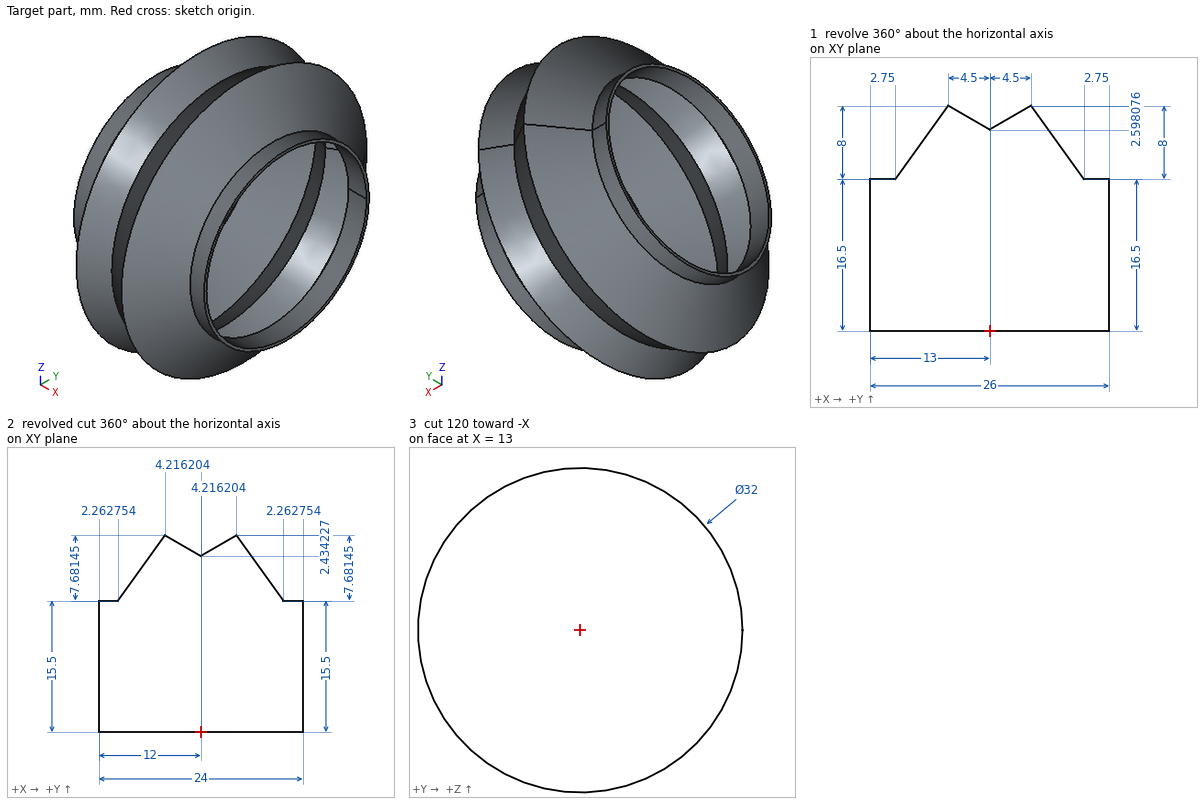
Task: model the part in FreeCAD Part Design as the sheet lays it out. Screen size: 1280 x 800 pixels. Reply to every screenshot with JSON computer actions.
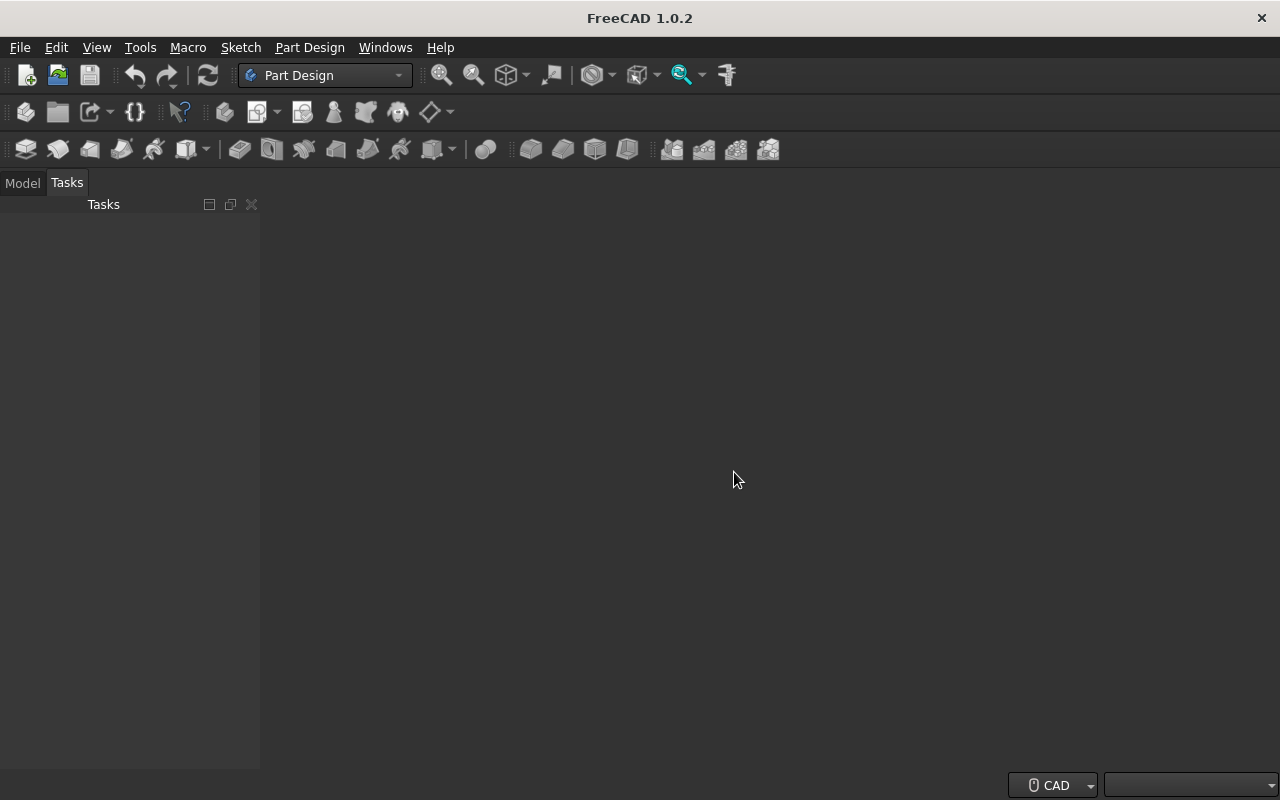
{"action": "key", "text": "ctrl+n"}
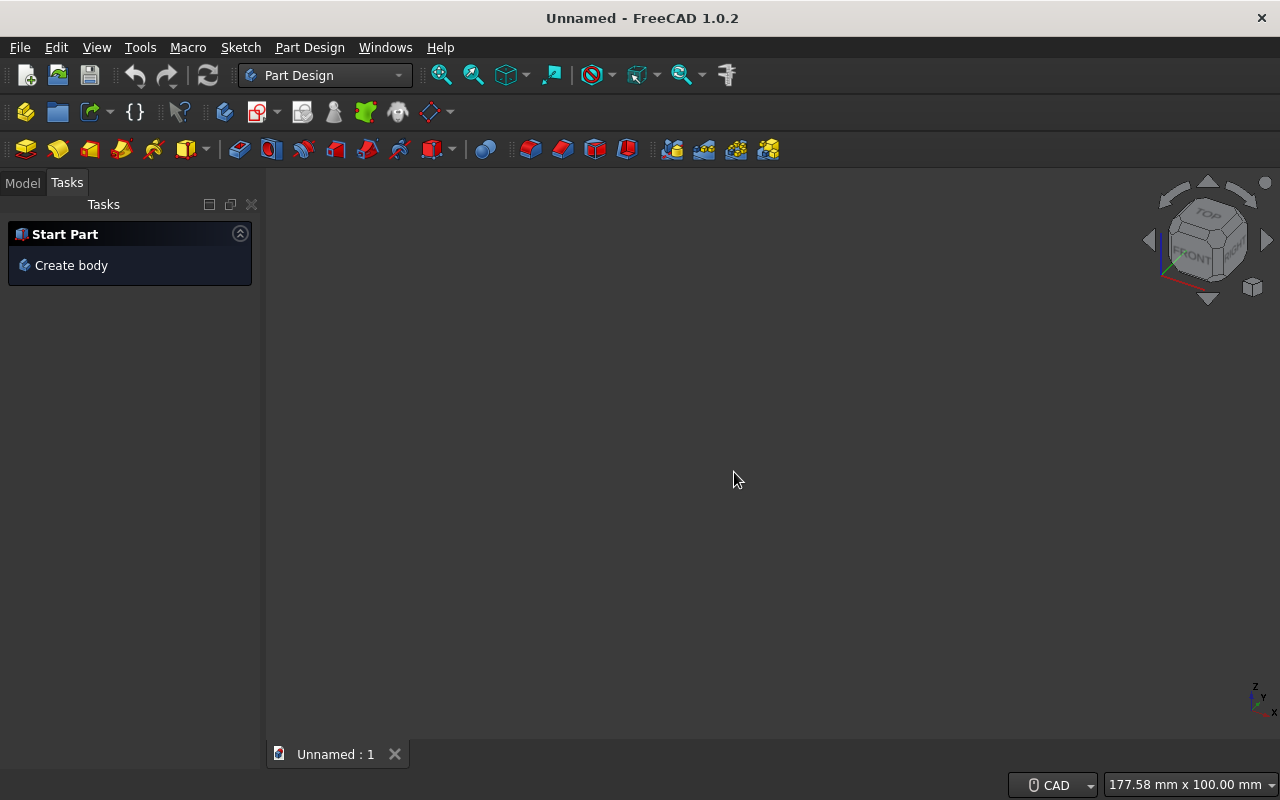
{"action": "left_click", "coordinate": [258, 112]}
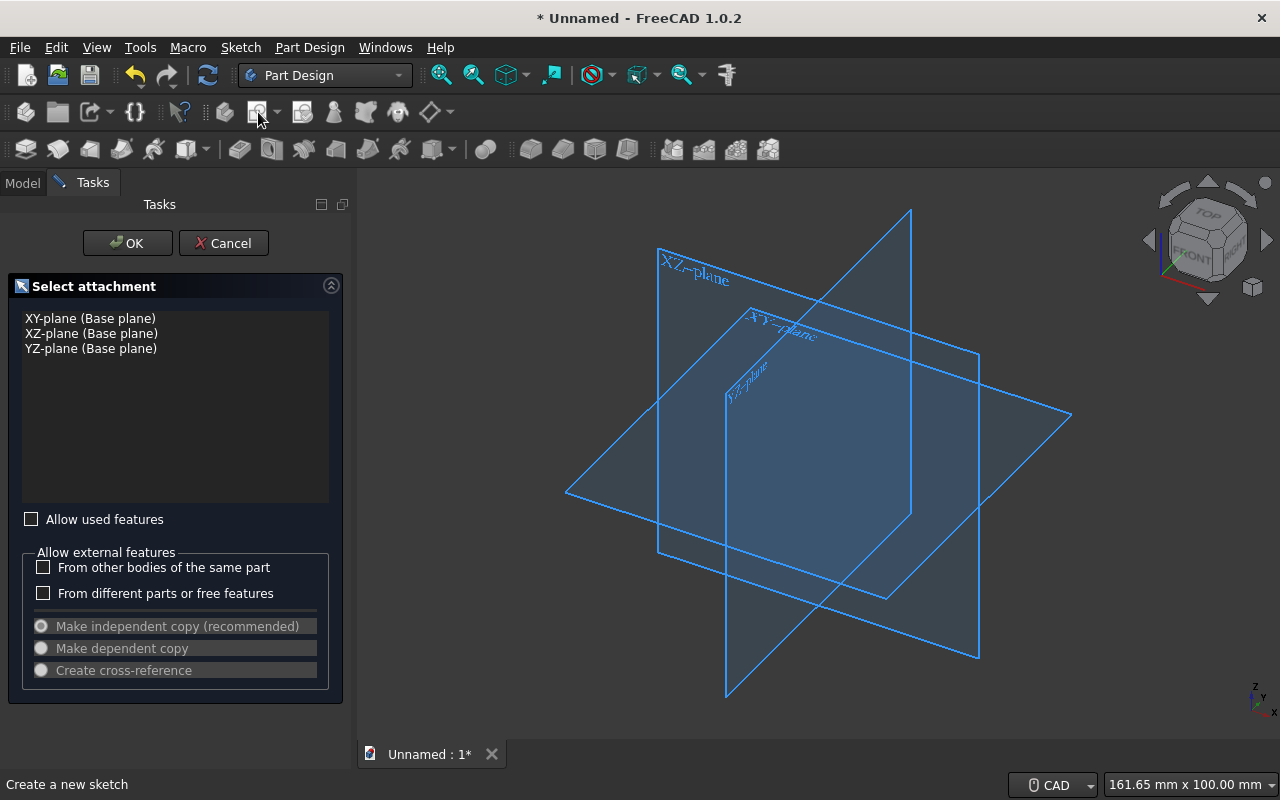
{"action": "left_click", "coordinate": [82, 318]}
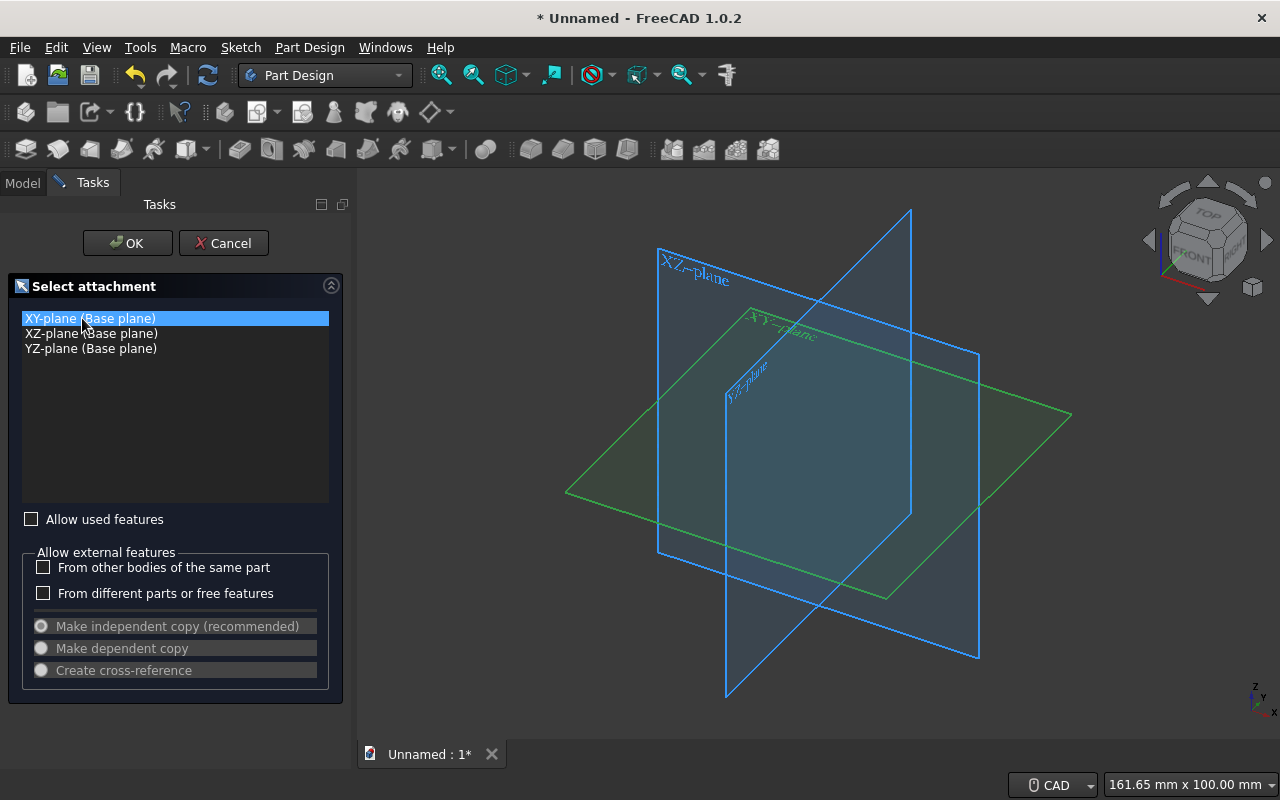
{"action": "left_click", "coordinate": [128, 243]}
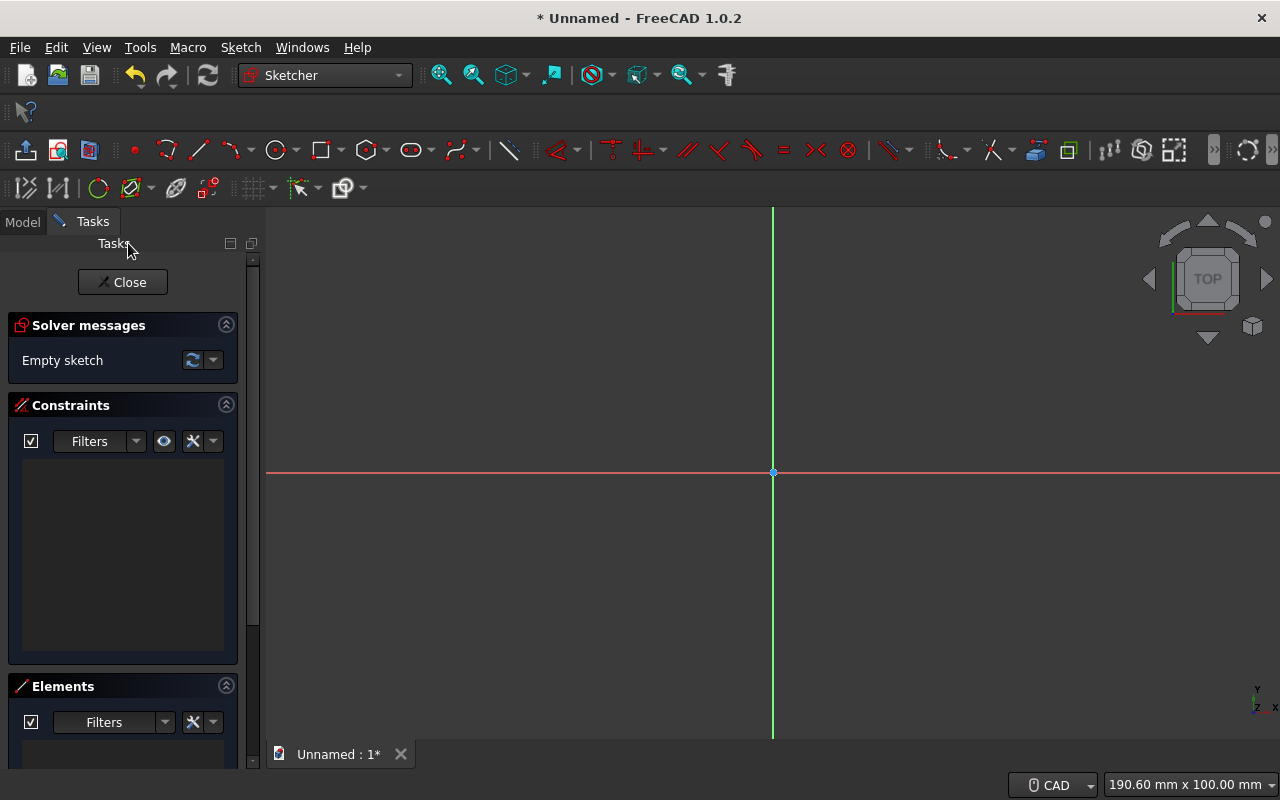
{"action": "scroll", "coordinate": [813, 370], "scroll_direction": "up", "scroll_amount": 5}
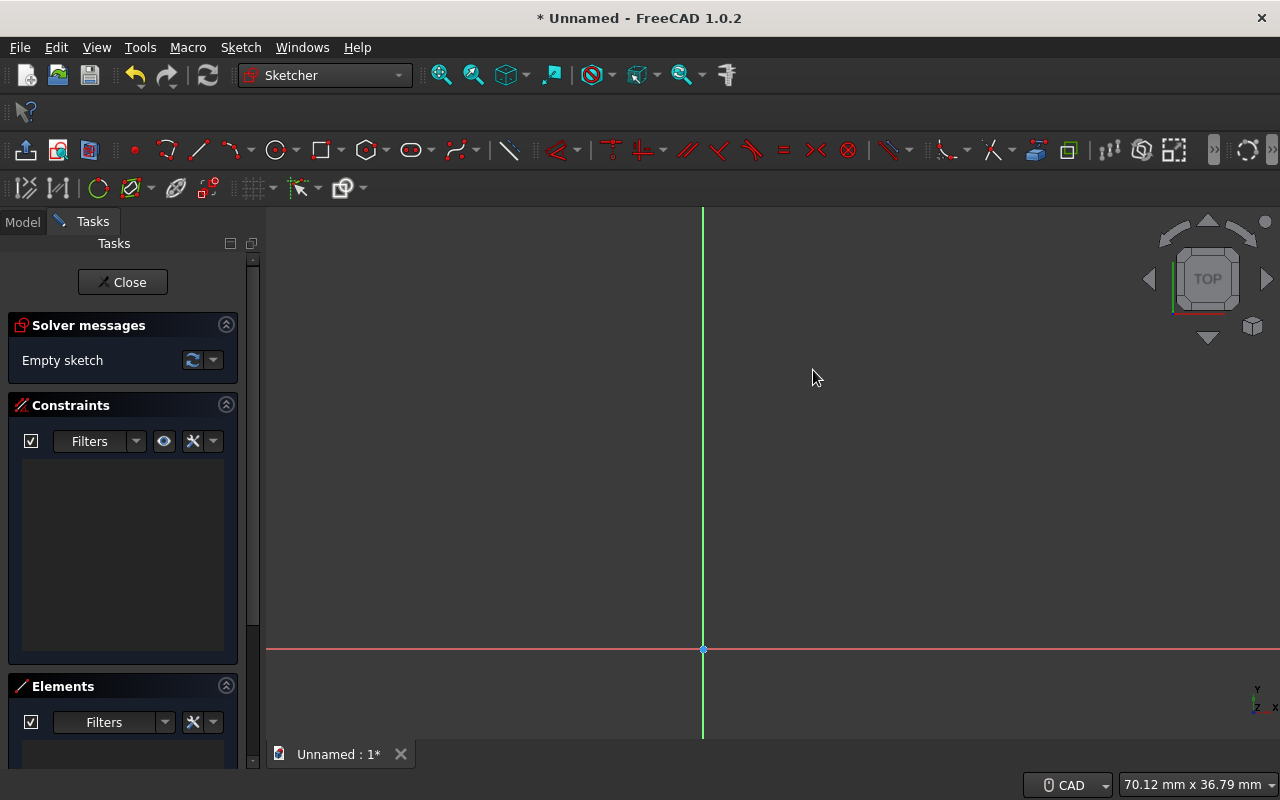
{"action": "key", "text": "g m"}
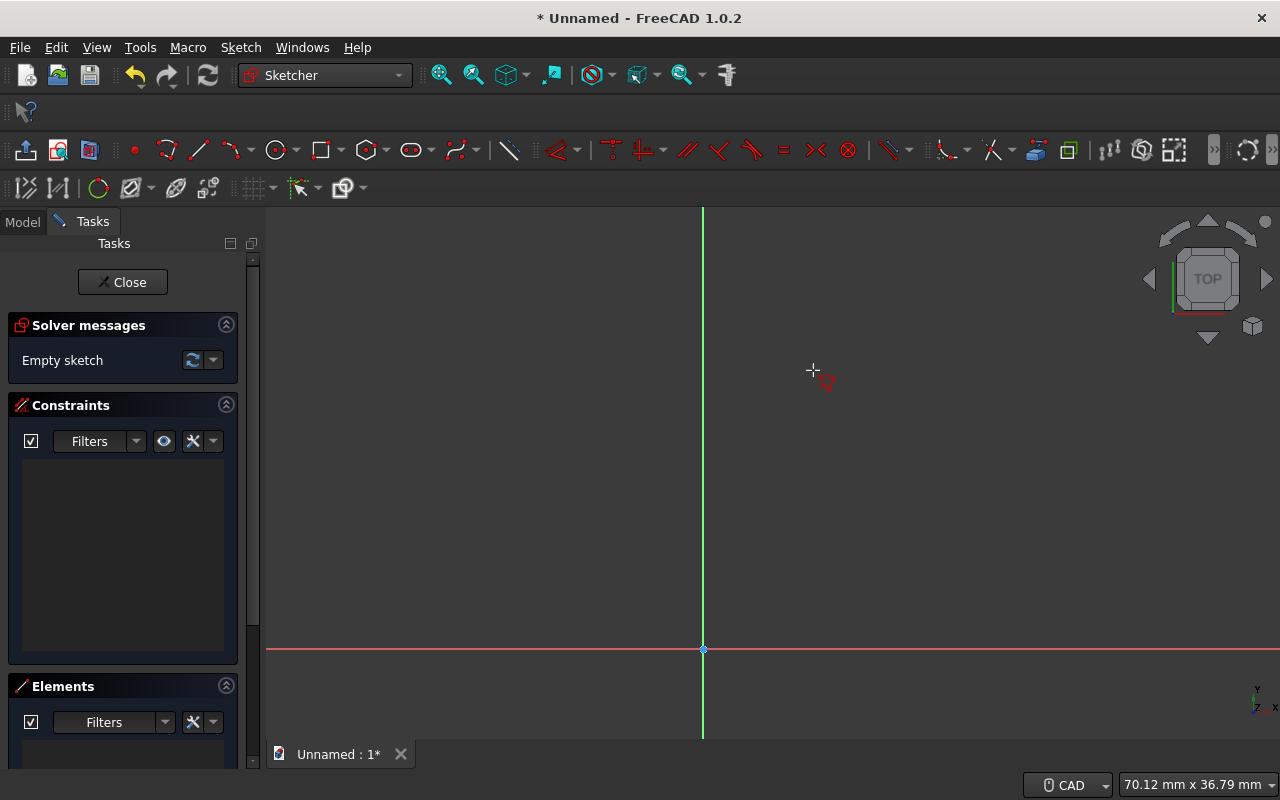
{"action": "left_click", "coordinate": [515, 649]}
{"action": "left_click", "coordinate": [891, 640]}
{"action": "left_click", "coordinate": [891, 411]}
{"action": "left_click", "coordinate": [852, 411]}
{"action": "left_click", "coordinate": [768, 295]}
{"action": "left_click", "coordinate": [703, 333]}
{"action": "left_click", "coordinate": [638, 295]}
{"action": "left_click", "coordinate": [555, 411]}
{"action": "left_click", "coordinate": [515, 411]}
{"action": "left_click", "coordinate": [515, 649]}
{"action": "key", "text": "Escape"}
{"action": "key", "text": "Escape"}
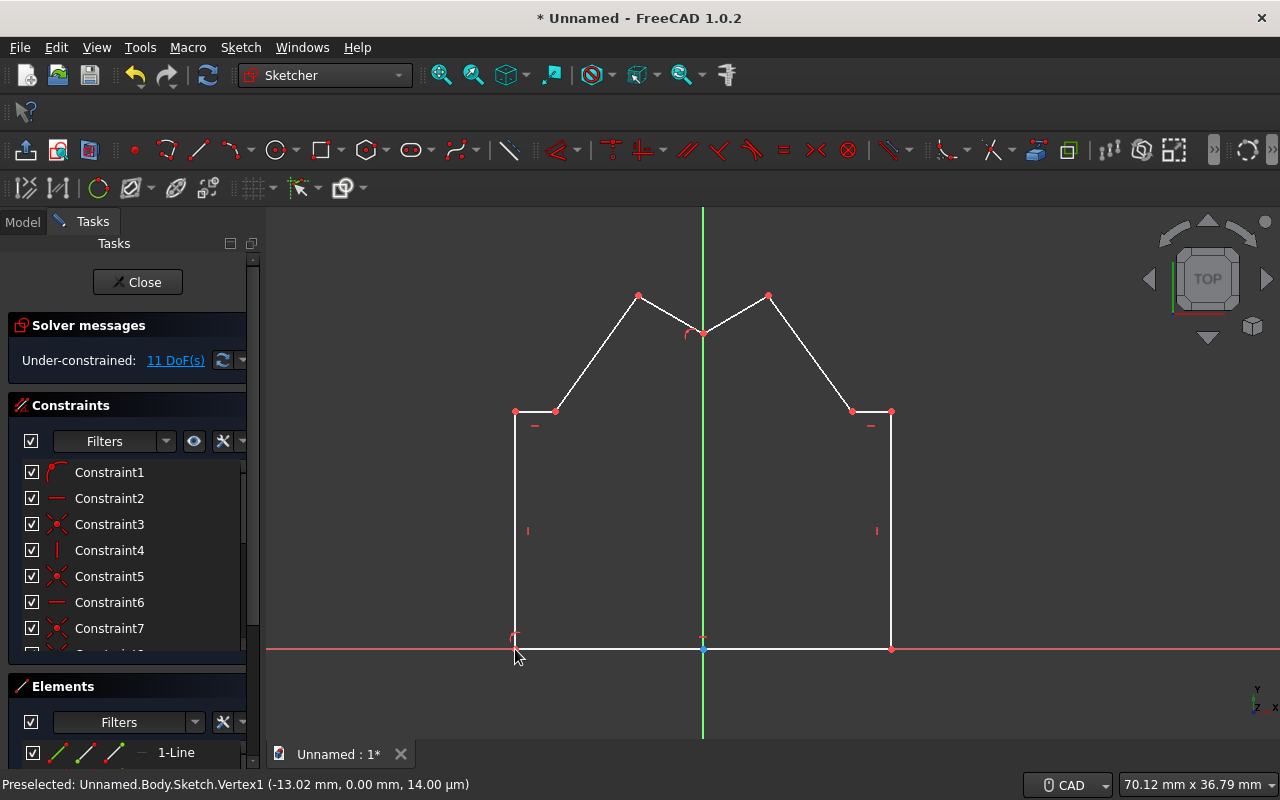
{"action": "left_click", "coordinate": [556, 150]}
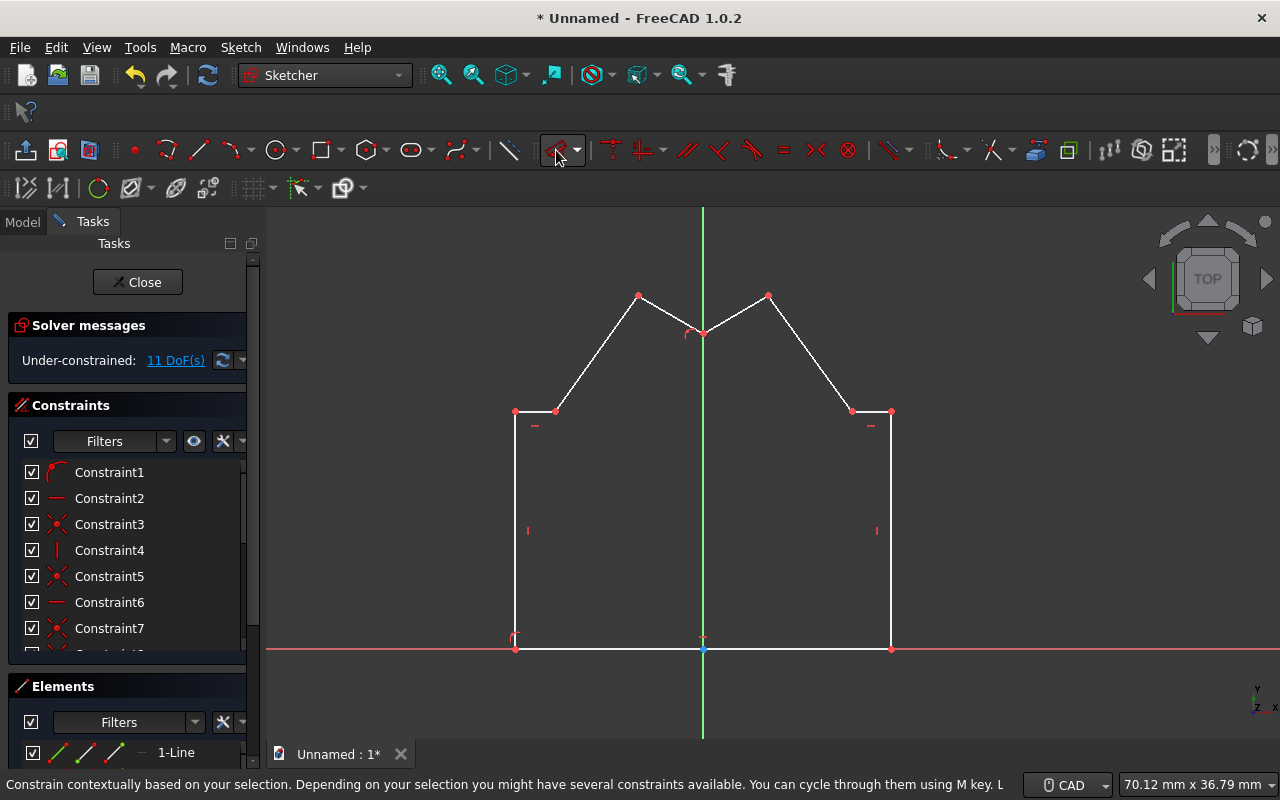
{"action": "left_click", "coordinate": [628, 649]}
{"action": "left_click", "coordinate": [617, 683]}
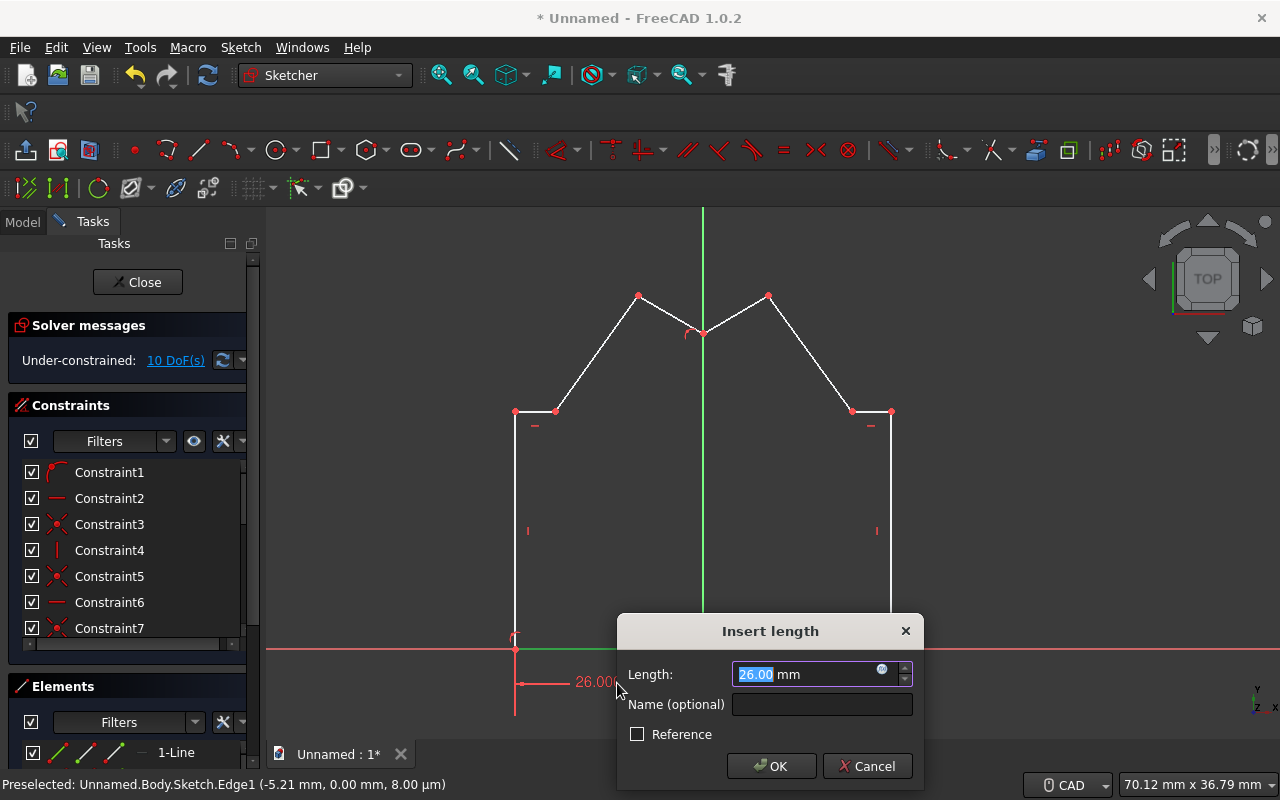
{"action": "type", "text": "26"}
{"action": "key", "text": "Return"}